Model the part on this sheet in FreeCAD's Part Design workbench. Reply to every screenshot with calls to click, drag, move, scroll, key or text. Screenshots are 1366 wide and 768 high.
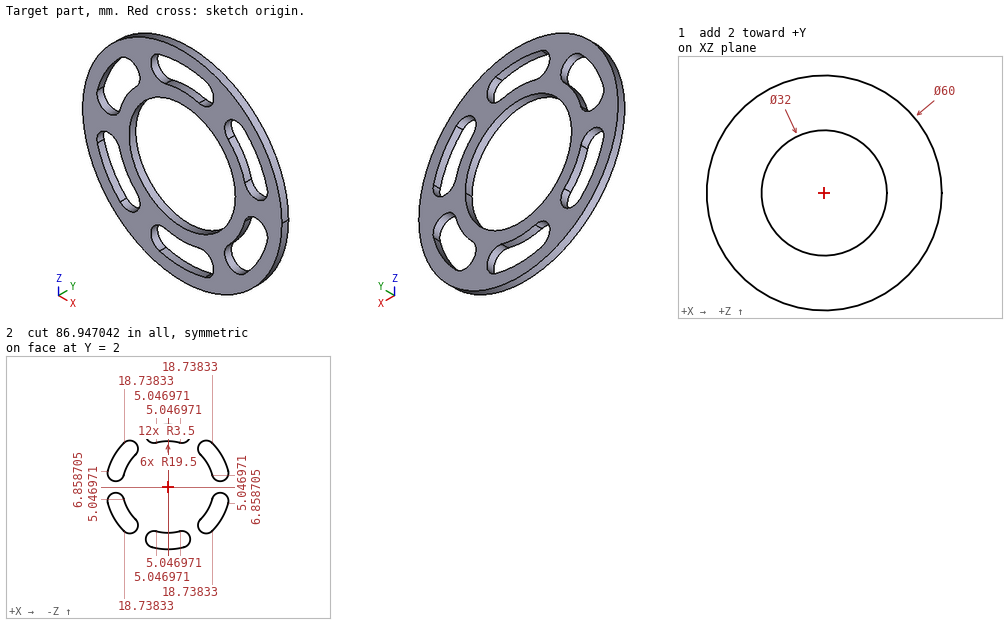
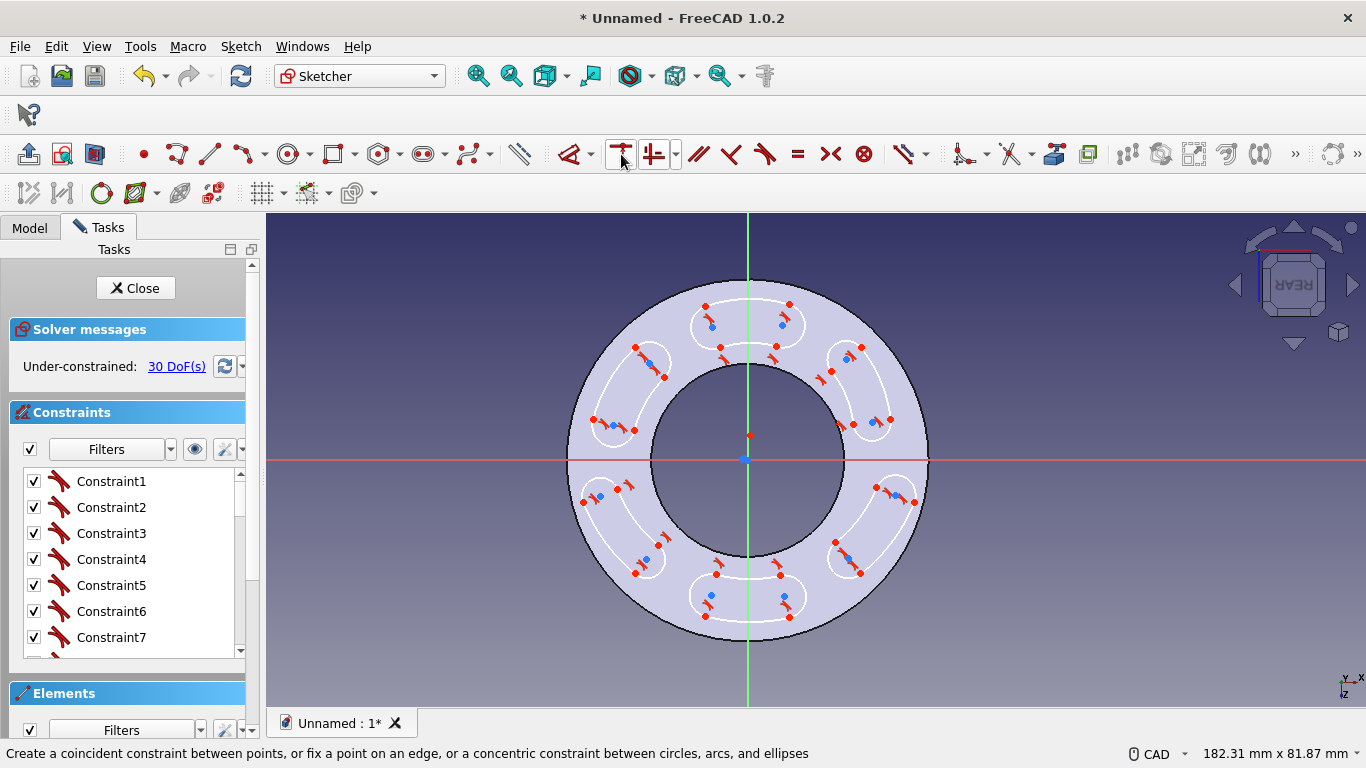
click(760, 343)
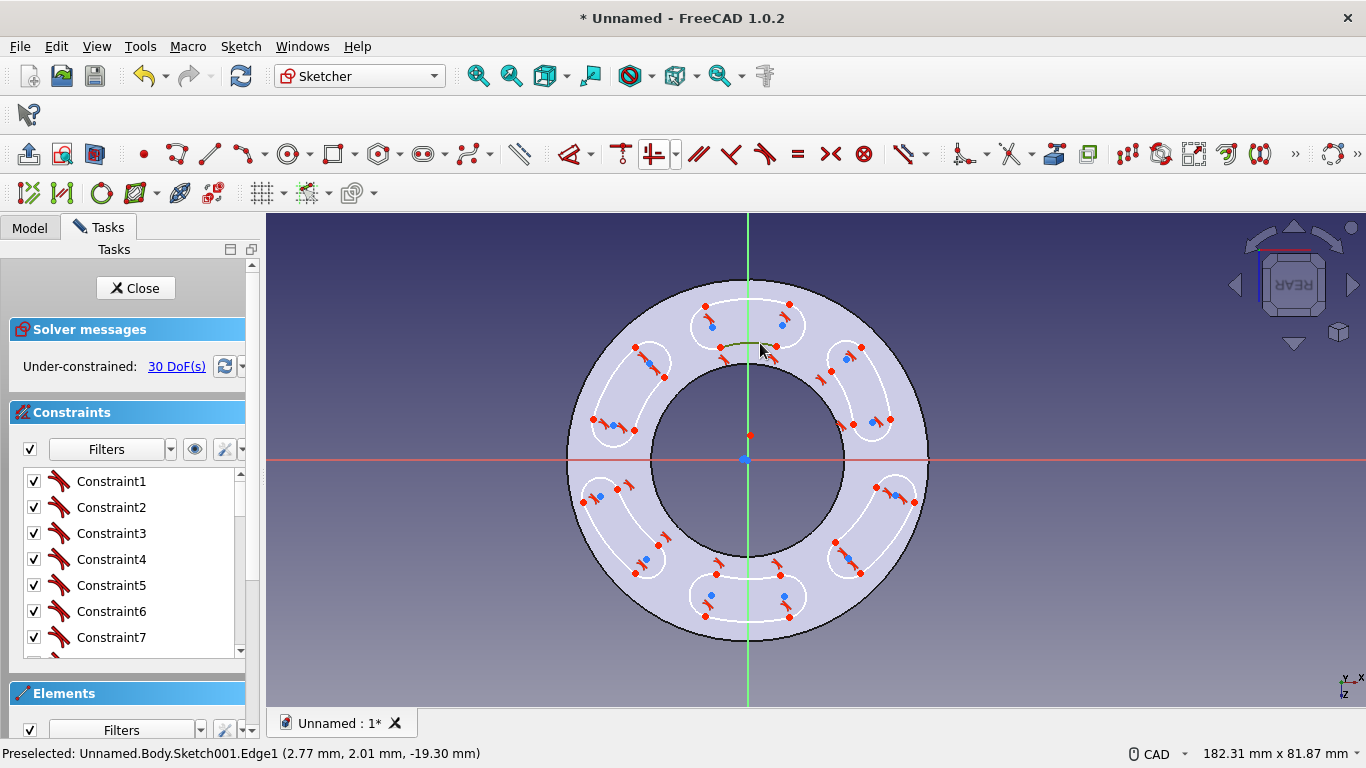
click(618, 367)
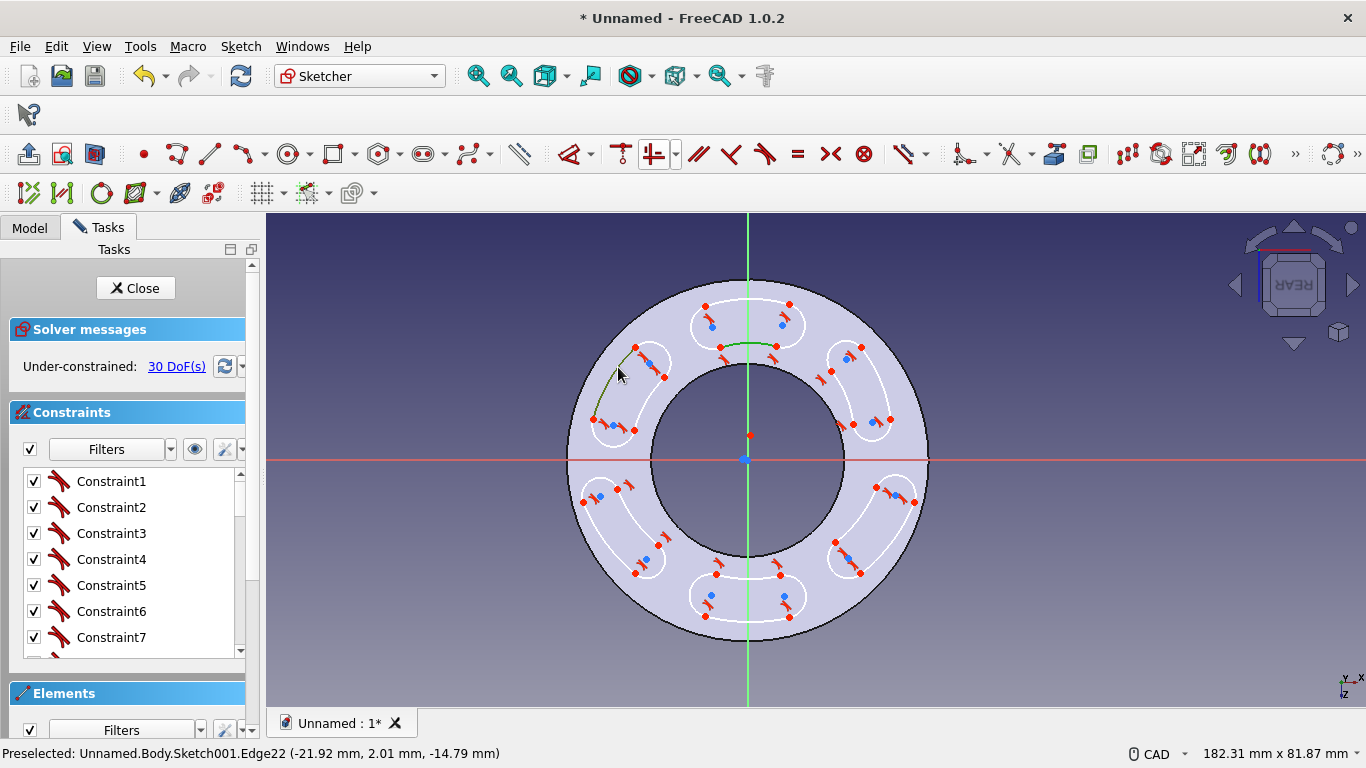
click(621, 154)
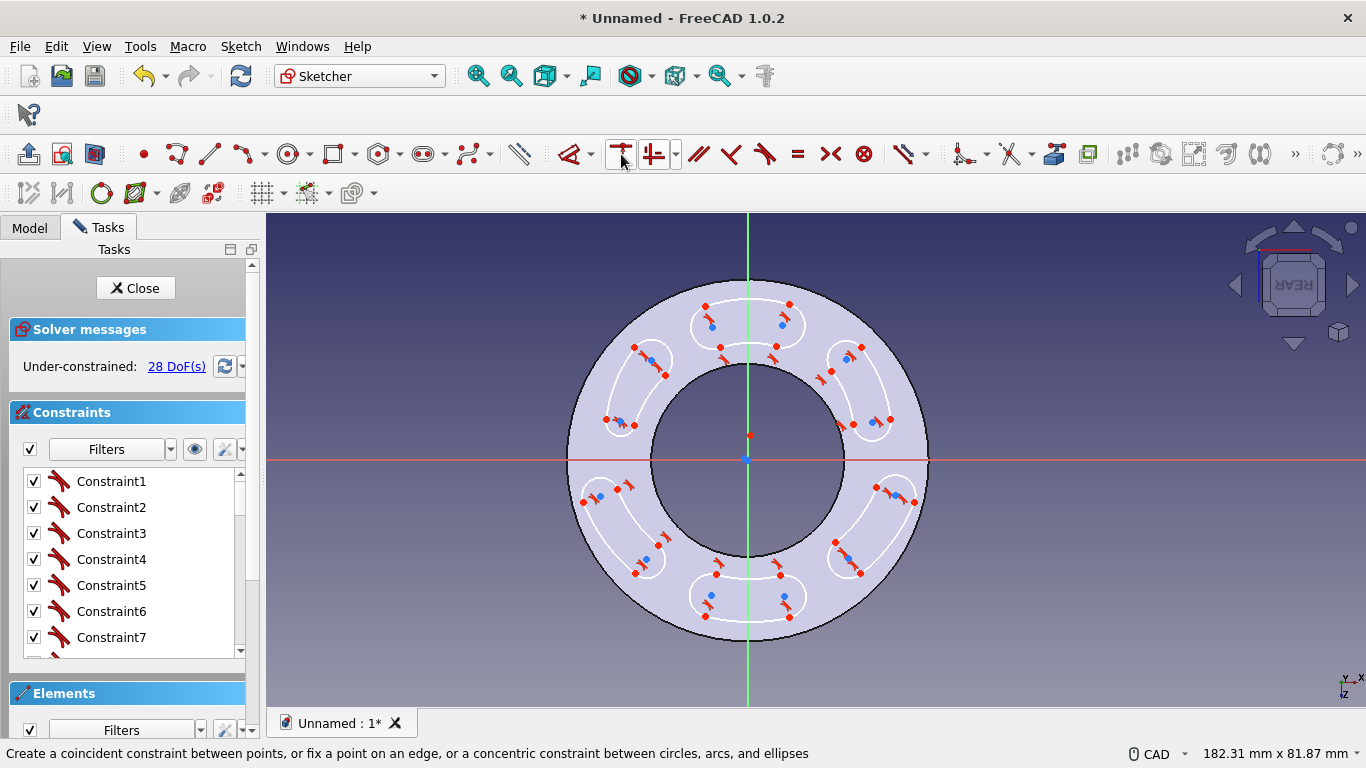
click(760, 343)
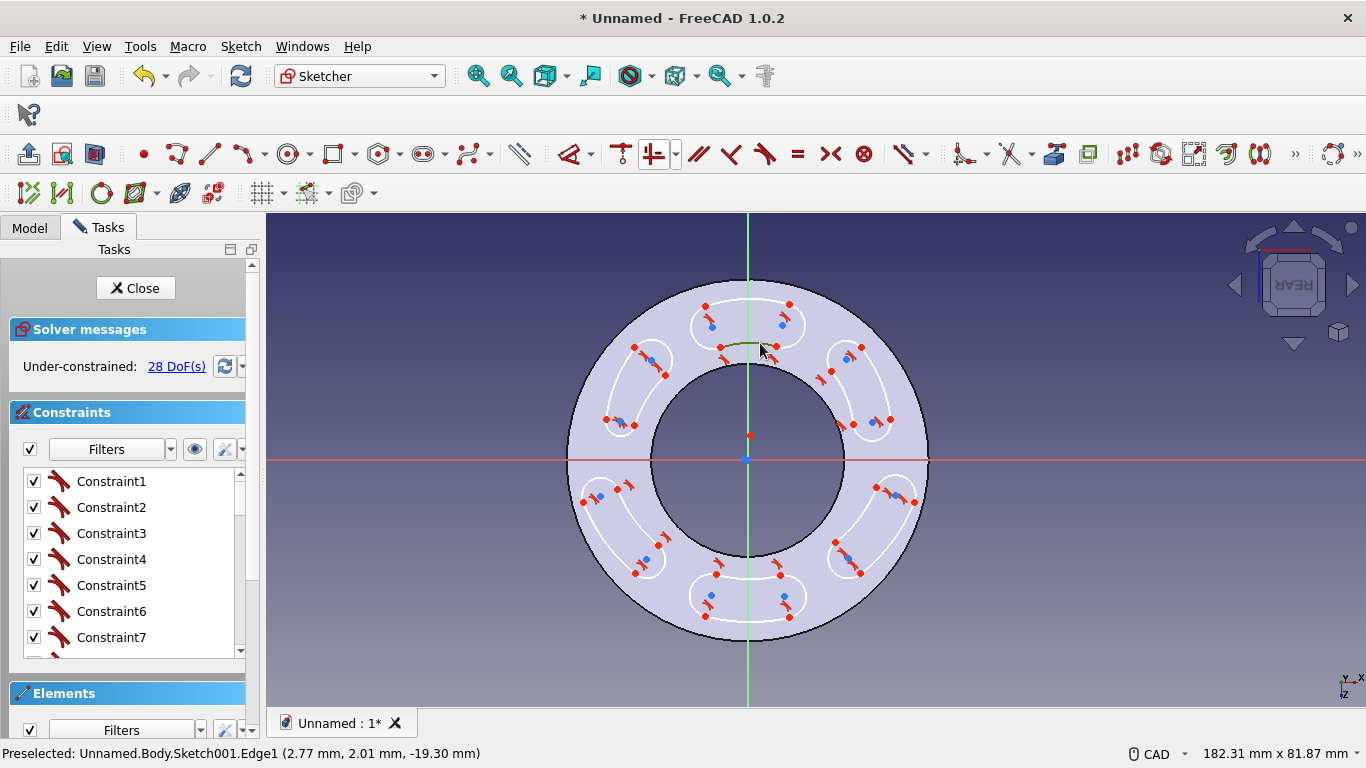
click(654, 389)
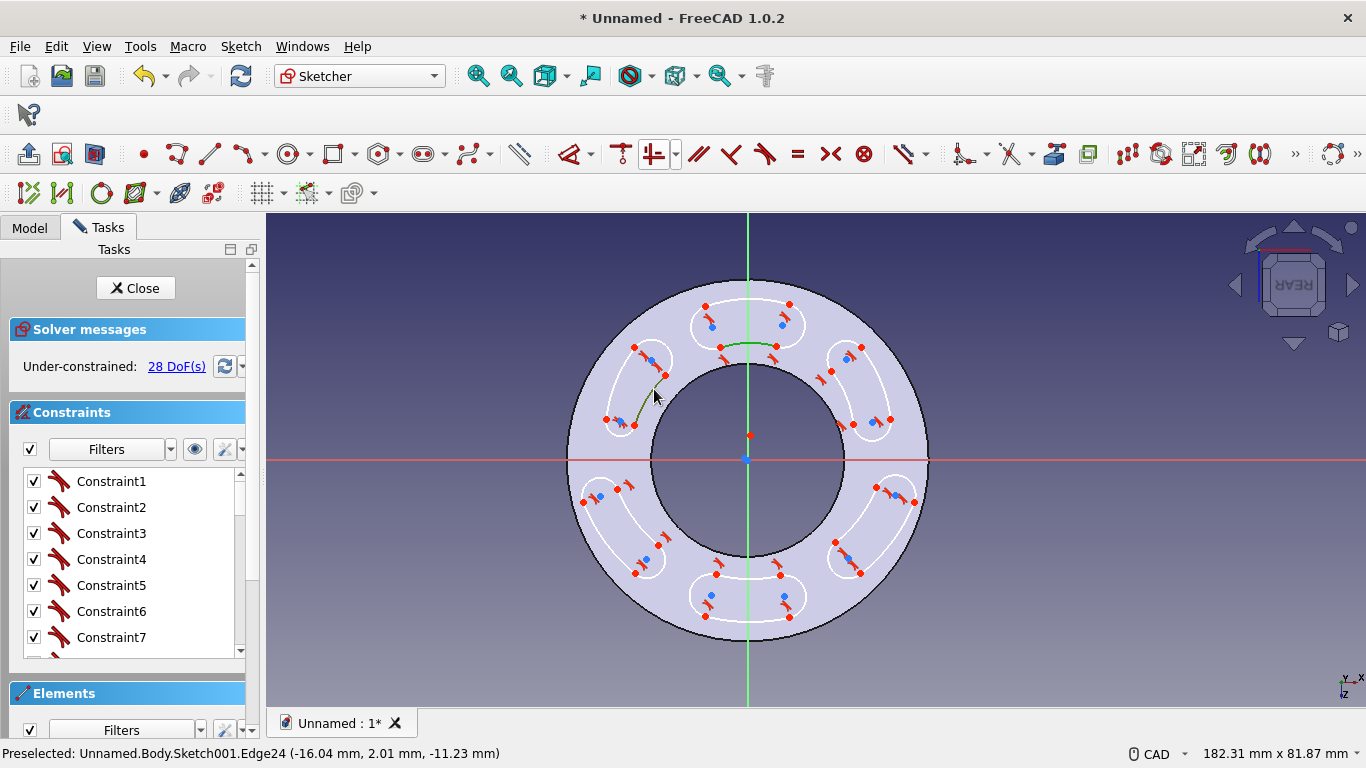
click(621, 154)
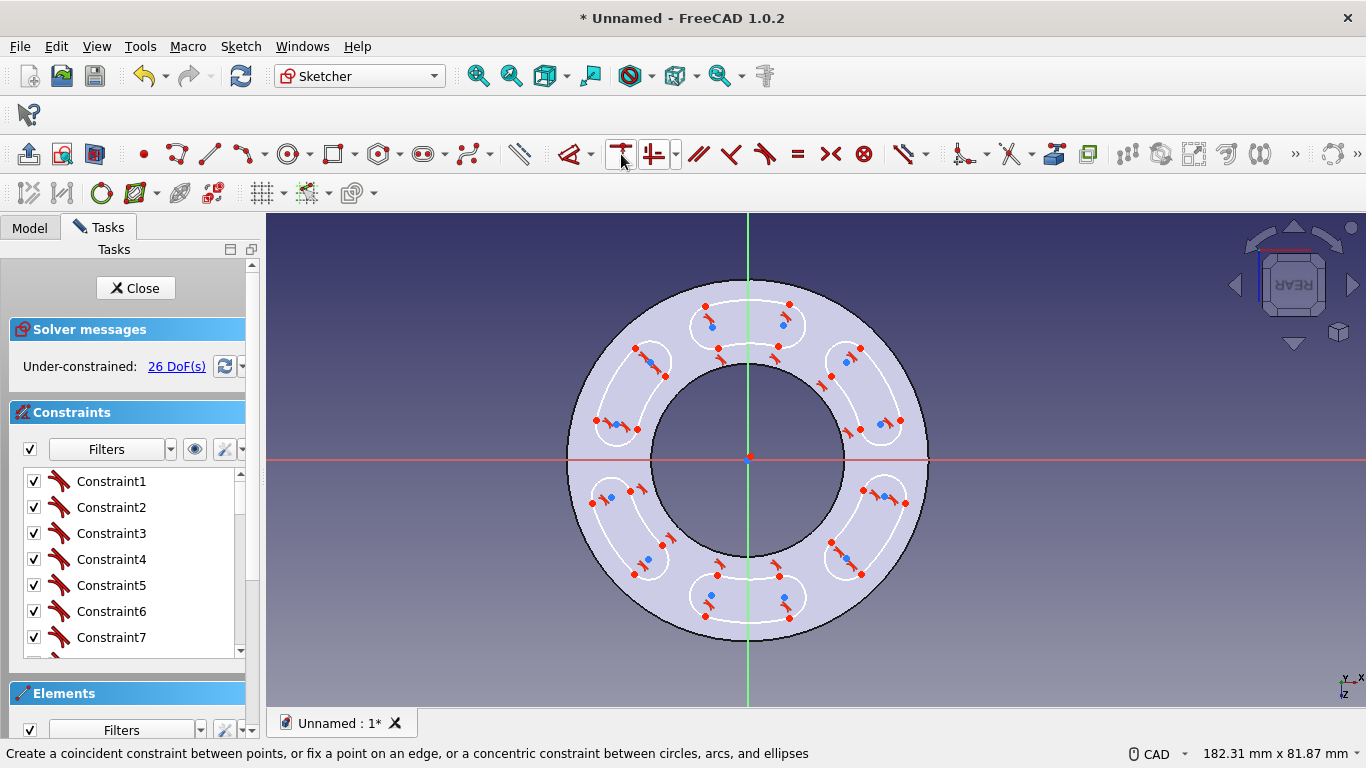
scroll(749, 458, up, 4)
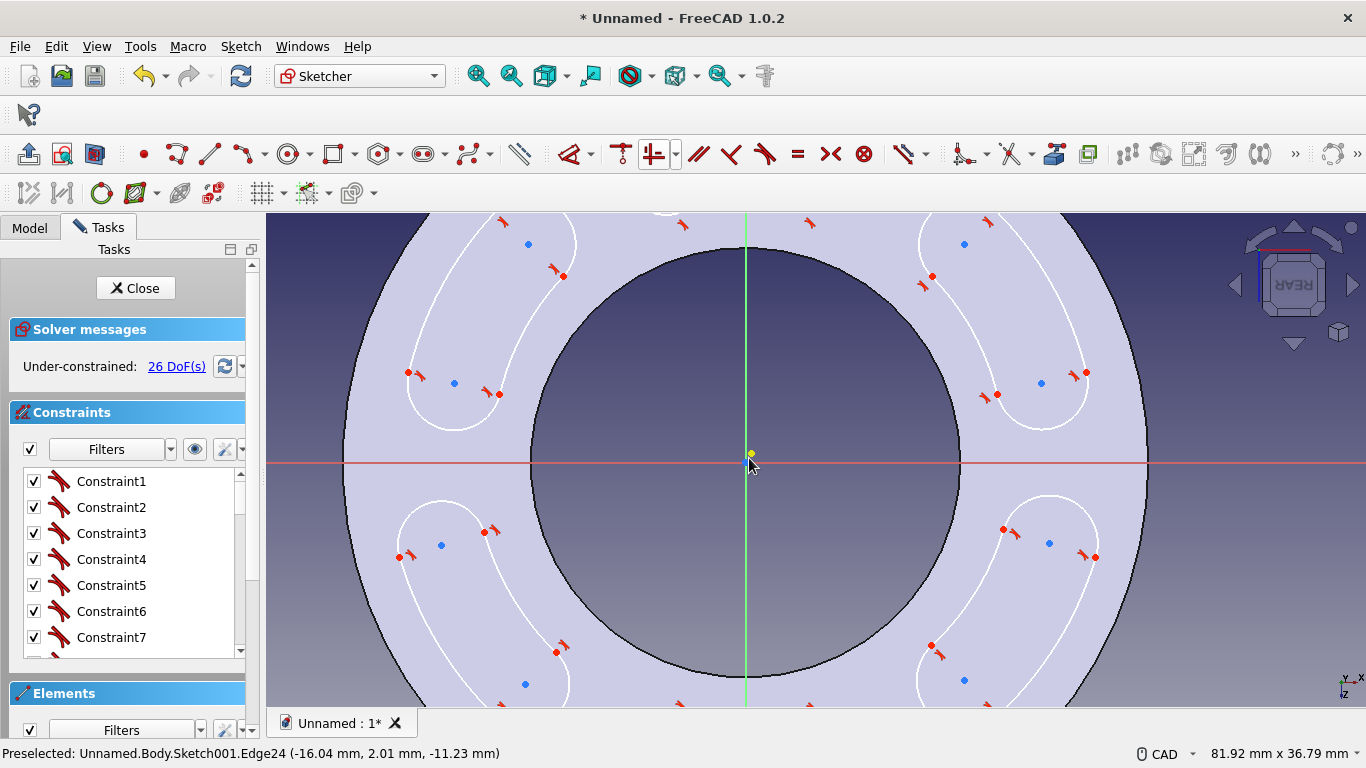
drag(736, 444, 762, 473)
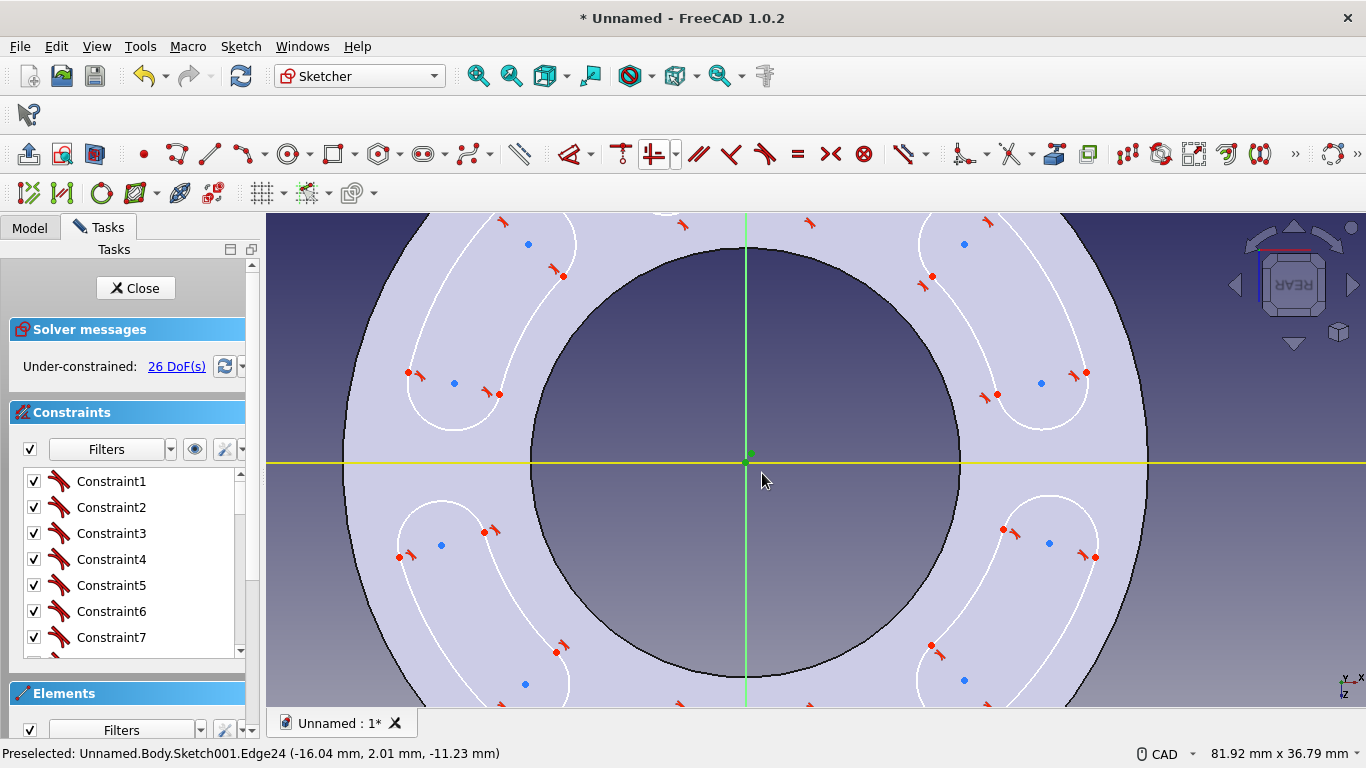
click(621, 154)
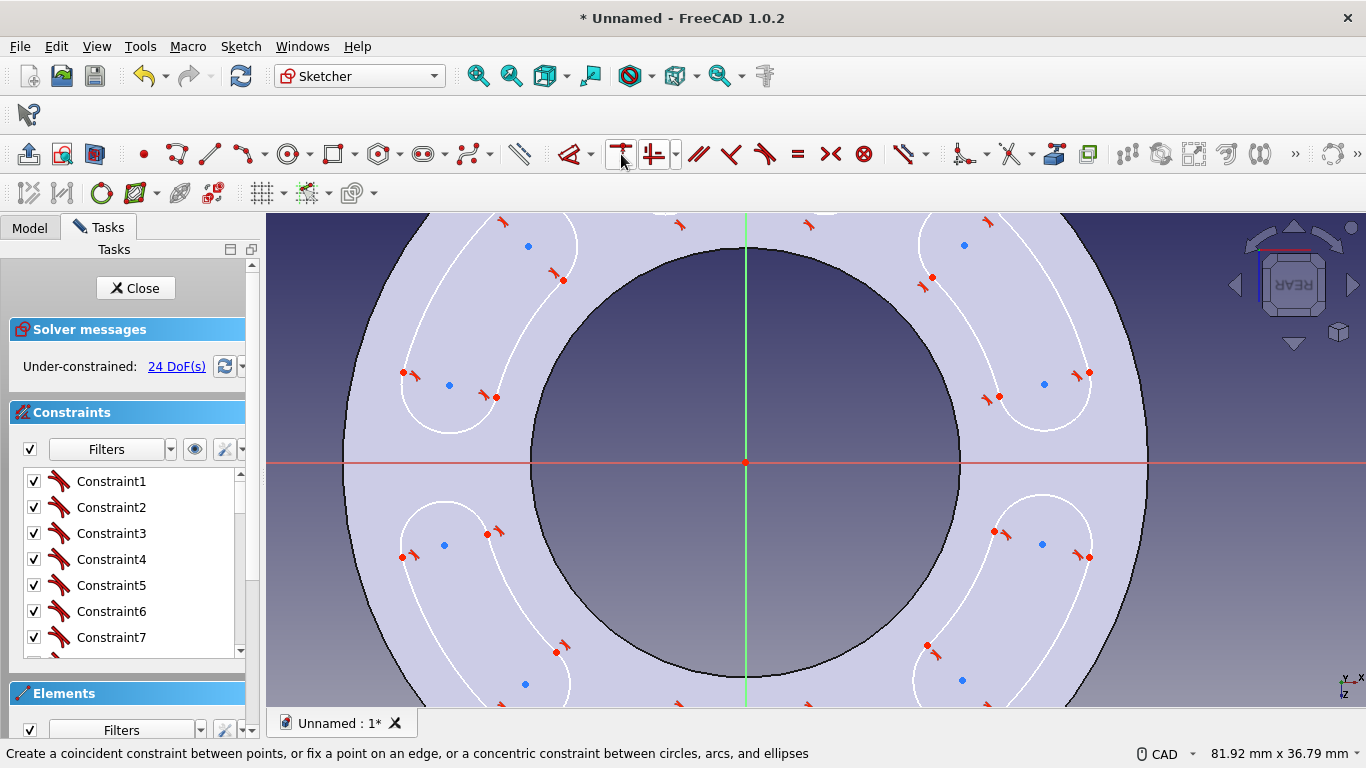
scroll(749, 458, down, 4)